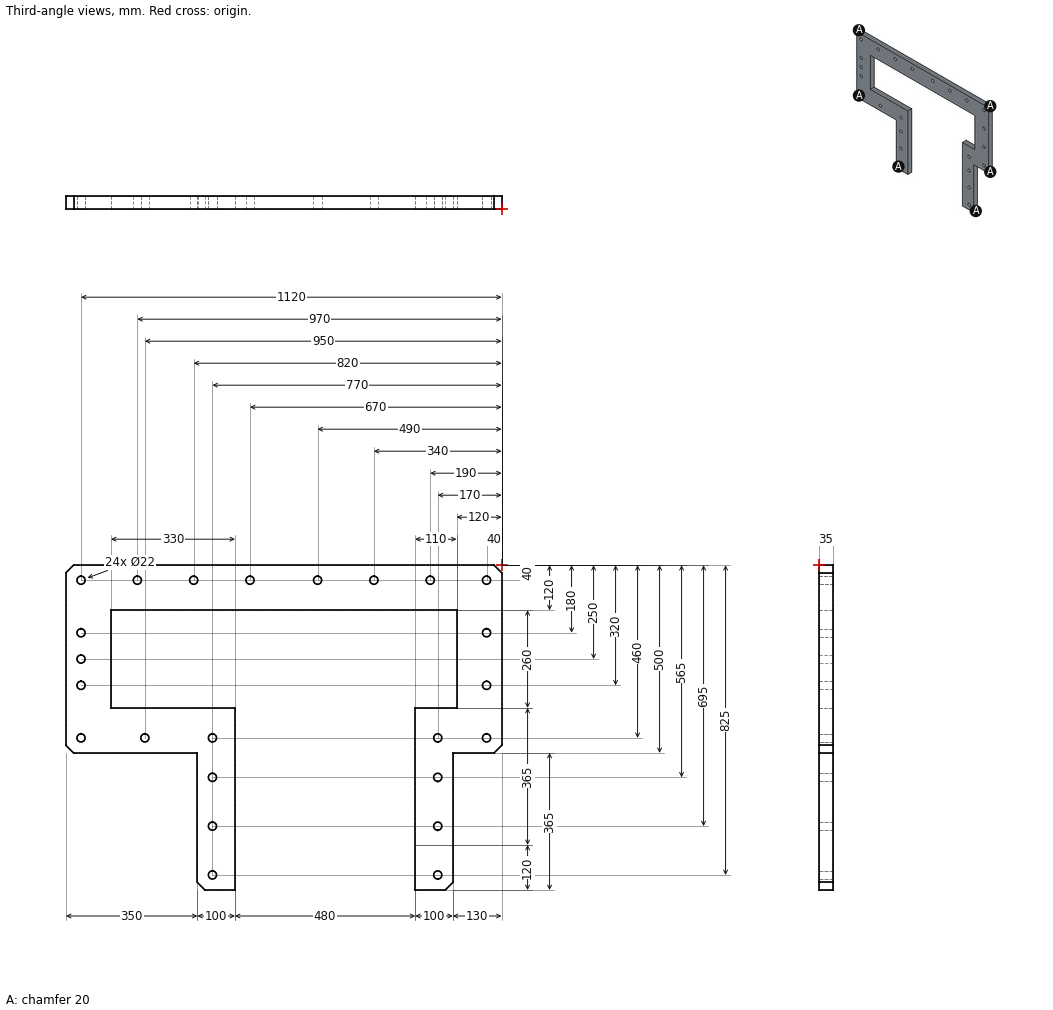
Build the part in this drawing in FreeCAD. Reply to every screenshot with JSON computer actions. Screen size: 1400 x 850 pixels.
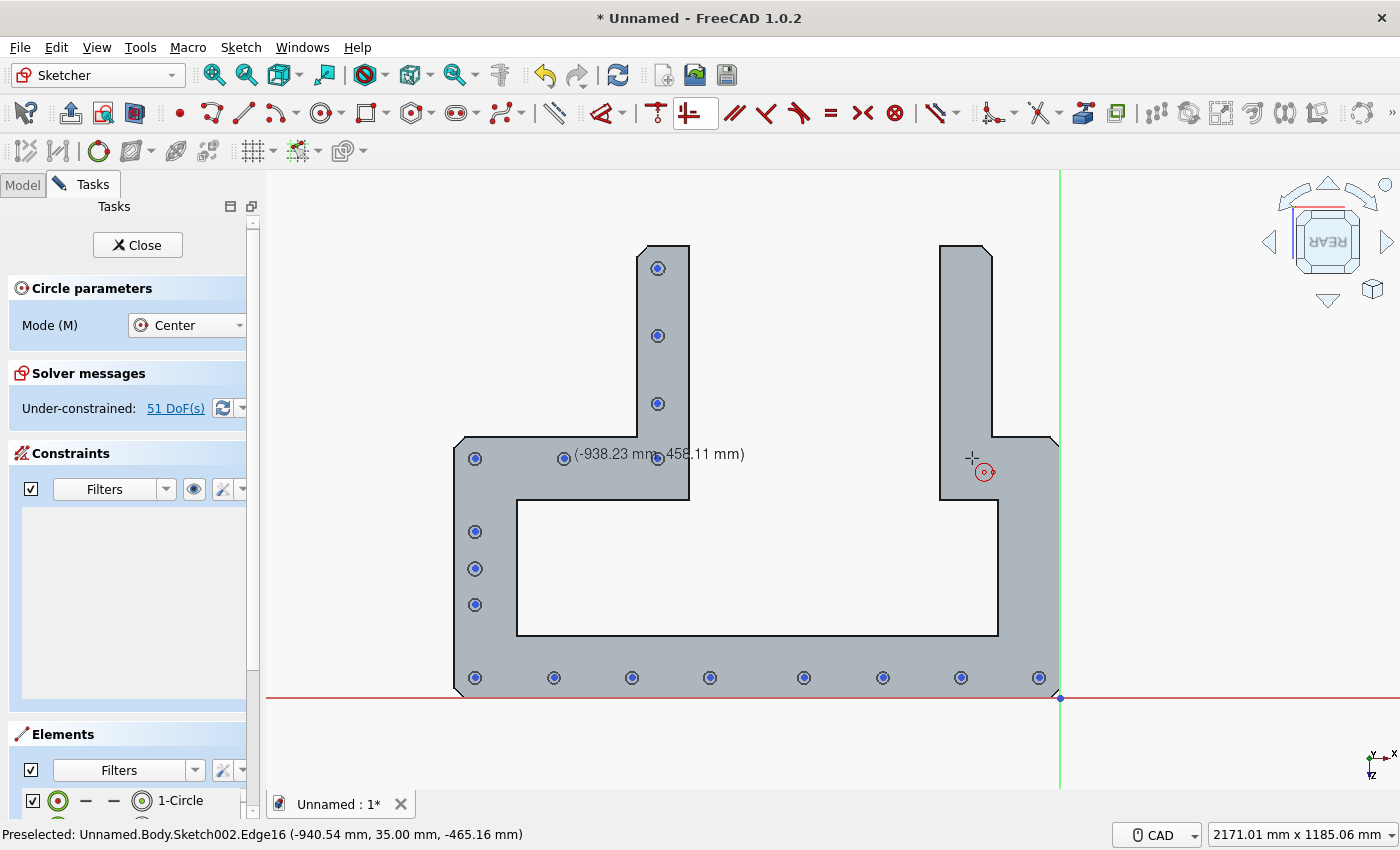
{"action": "left_click", "coordinate": [972, 458]}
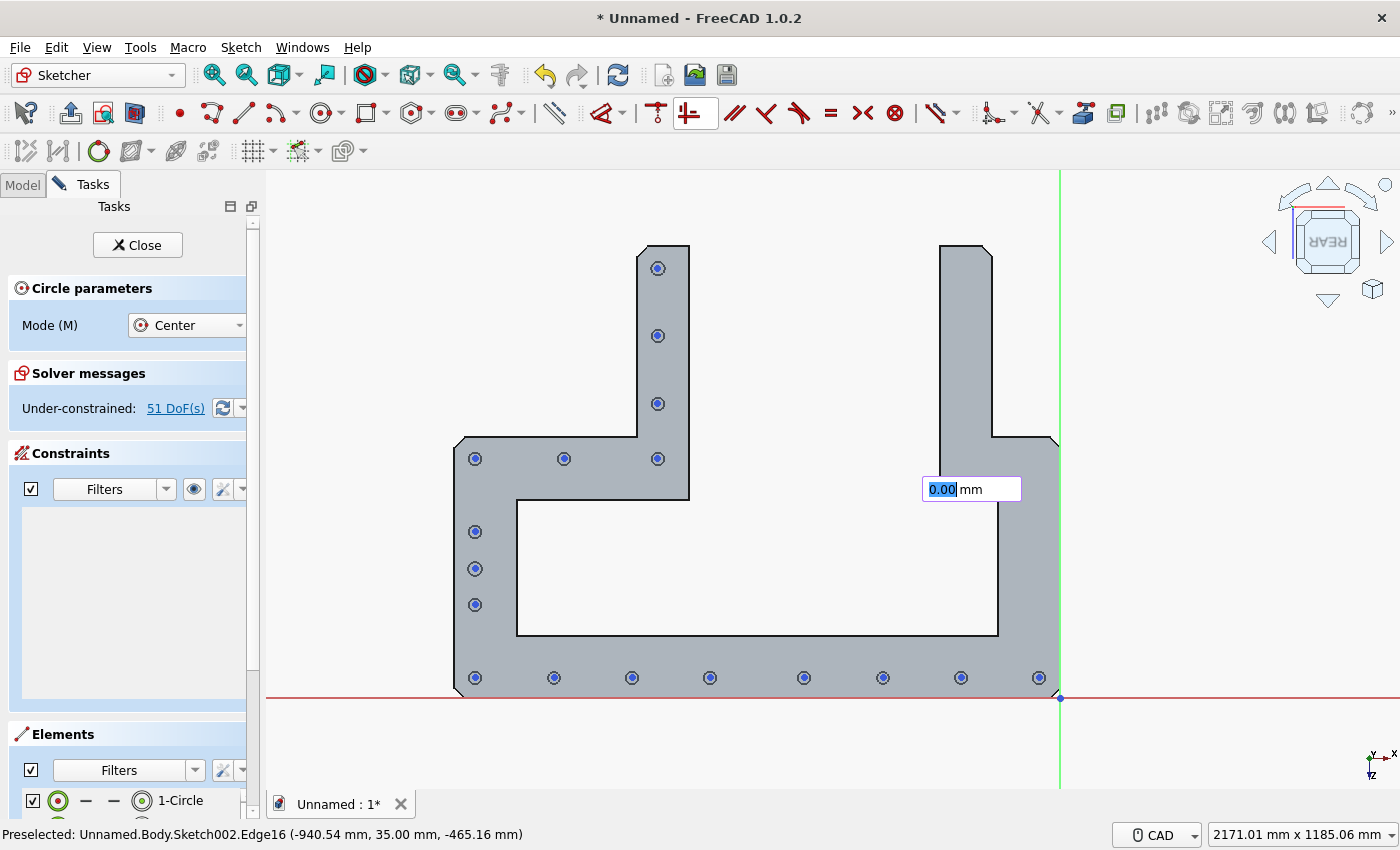
{"action": "scroll", "coordinate": [976, 454], "scroll_direction": "up", "scroll_amount": 6}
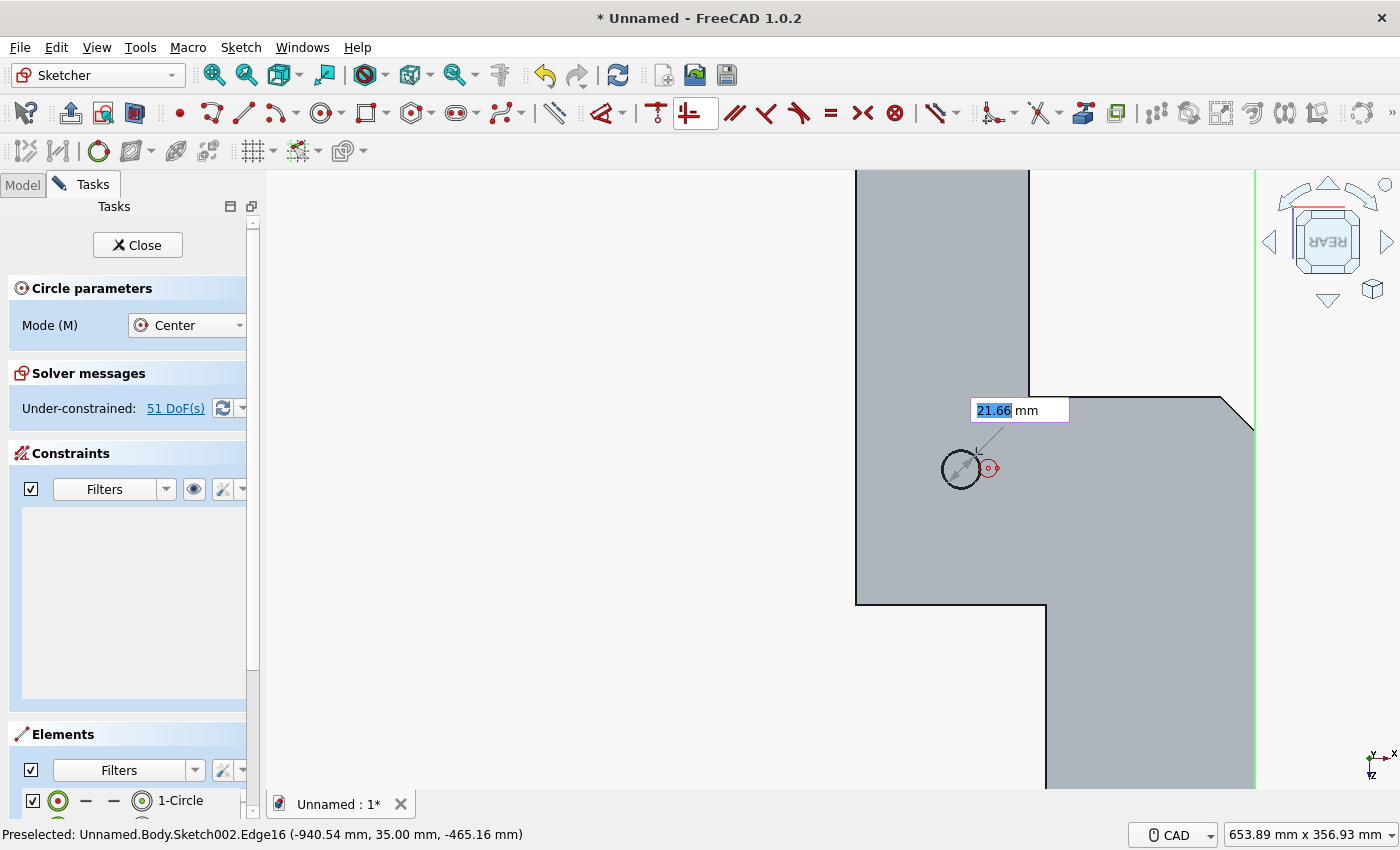
{"action": "left_click", "coordinate": [973, 453]}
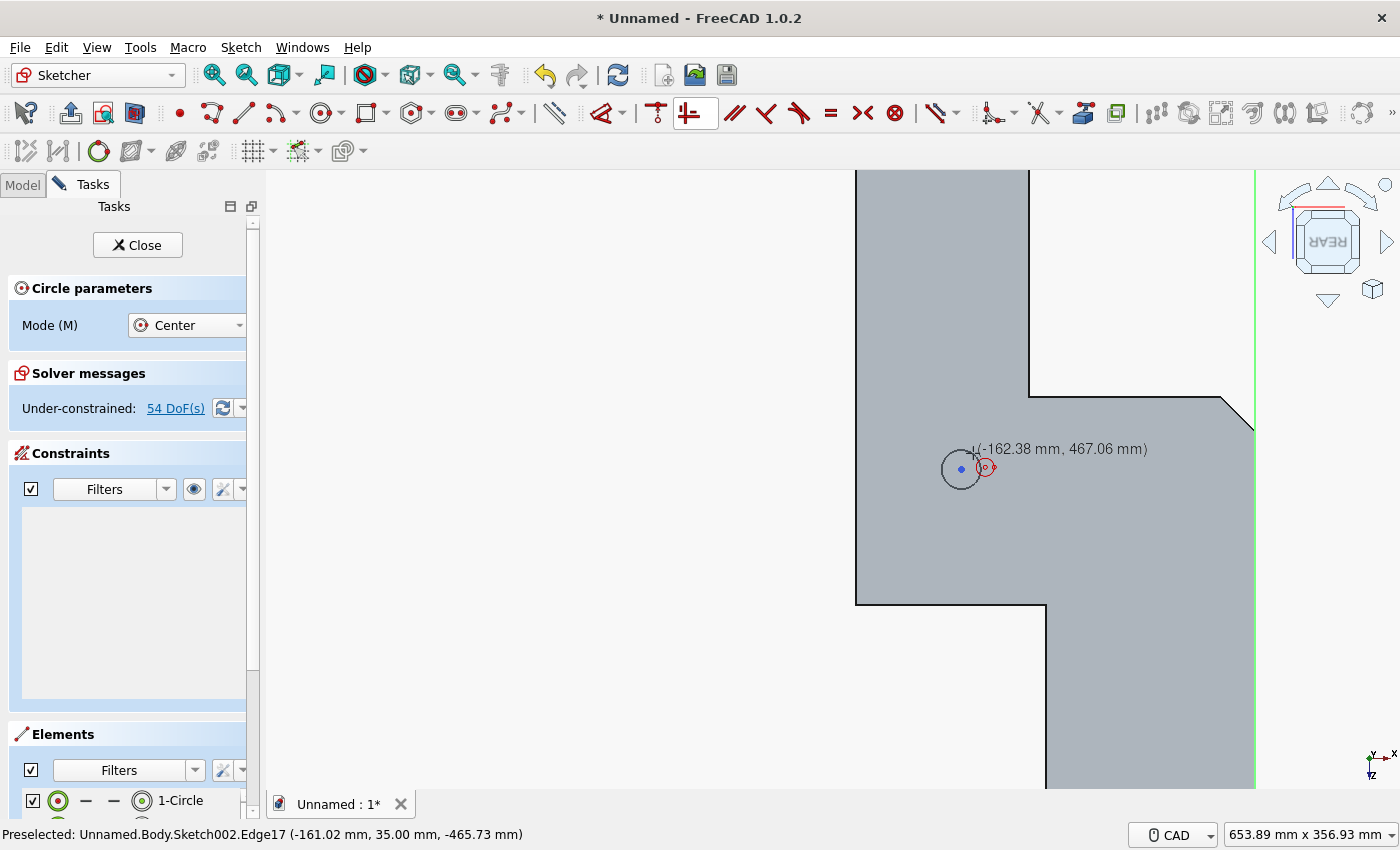
{"action": "scroll", "coordinate": [976, 454], "scroll_direction": "down", "scroll_amount": 6}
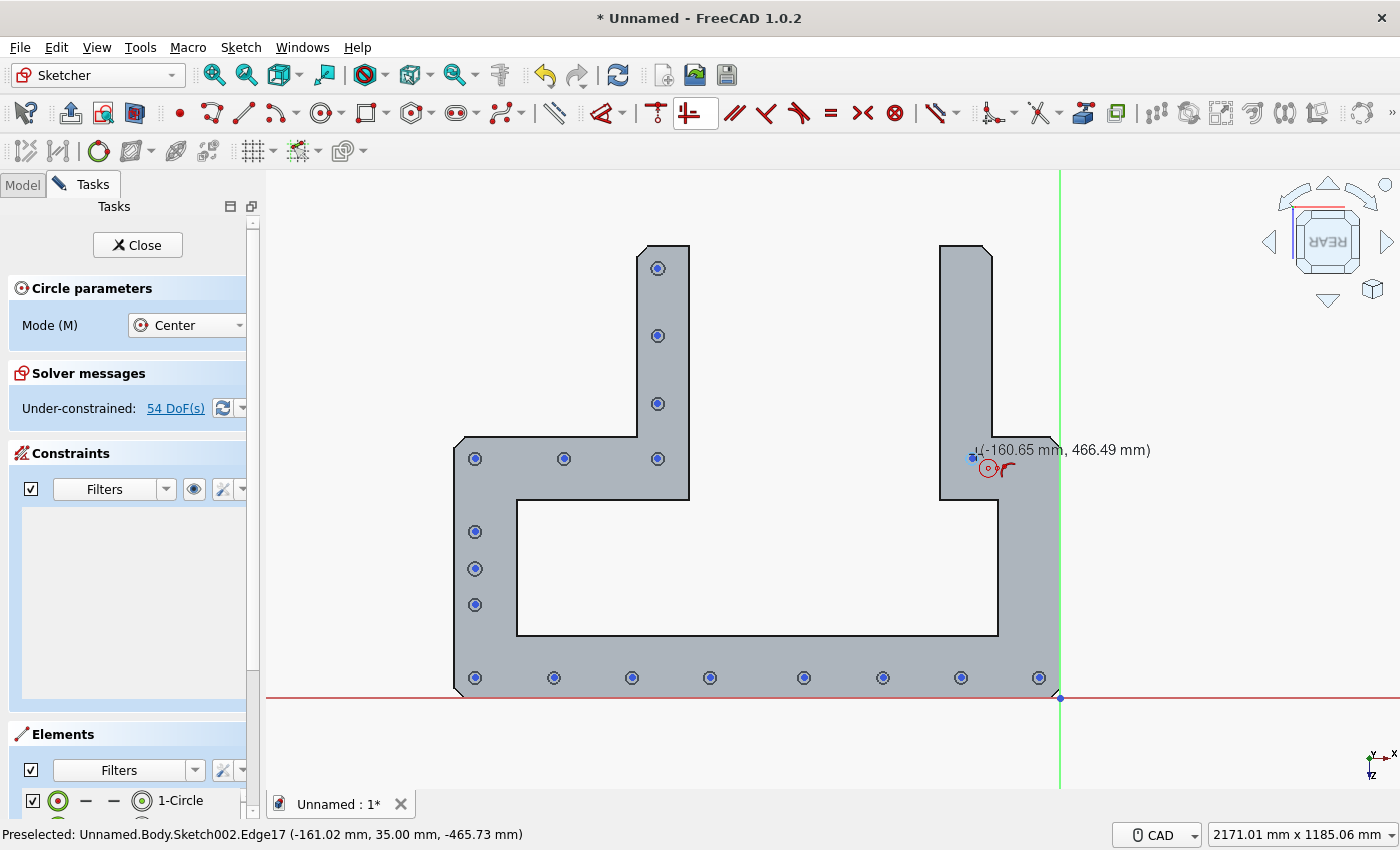
{"action": "left_click", "coordinate": [972, 403]}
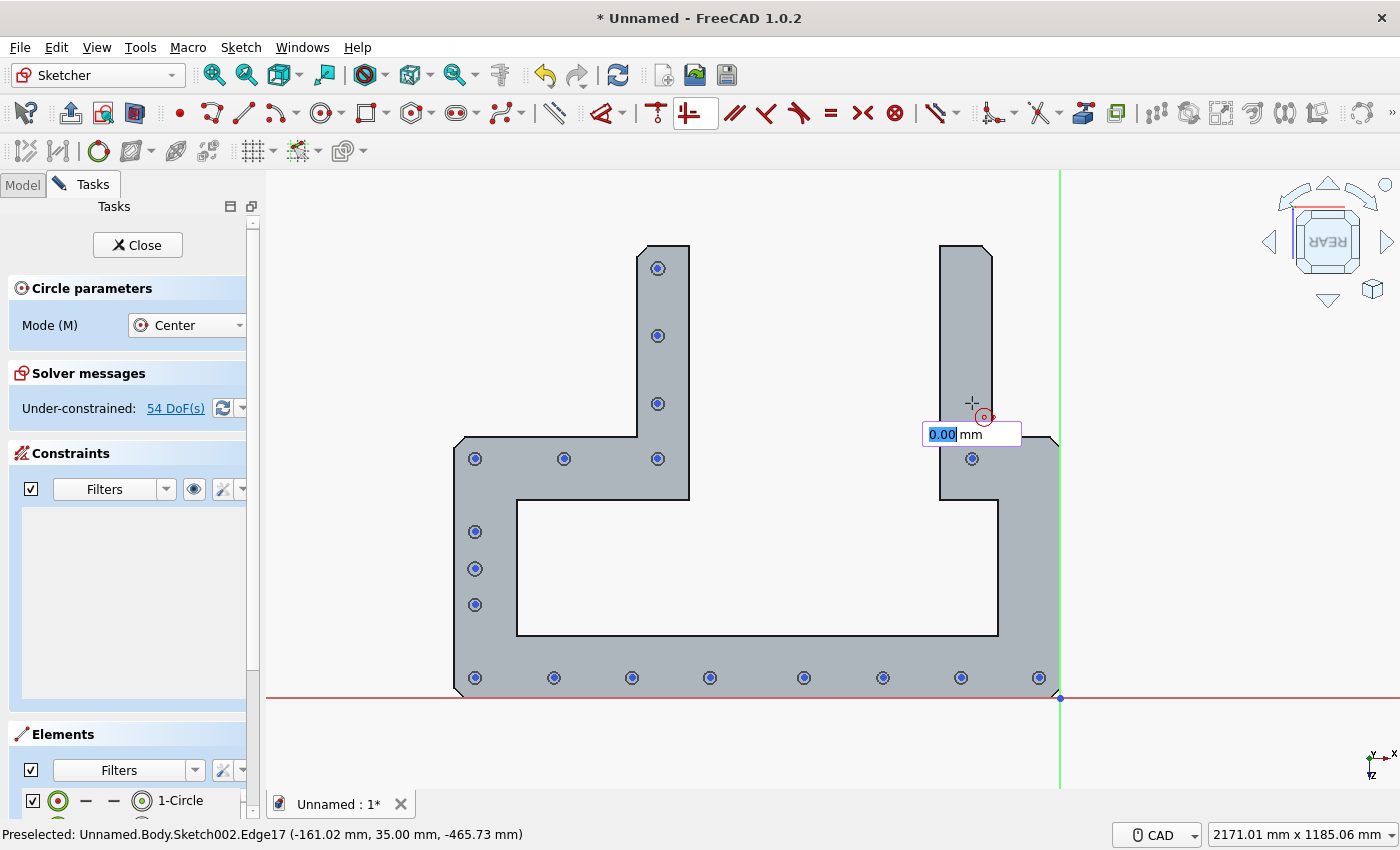
{"action": "scroll", "coordinate": [976, 399], "scroll_direction": "up", "scroll_amount": 6}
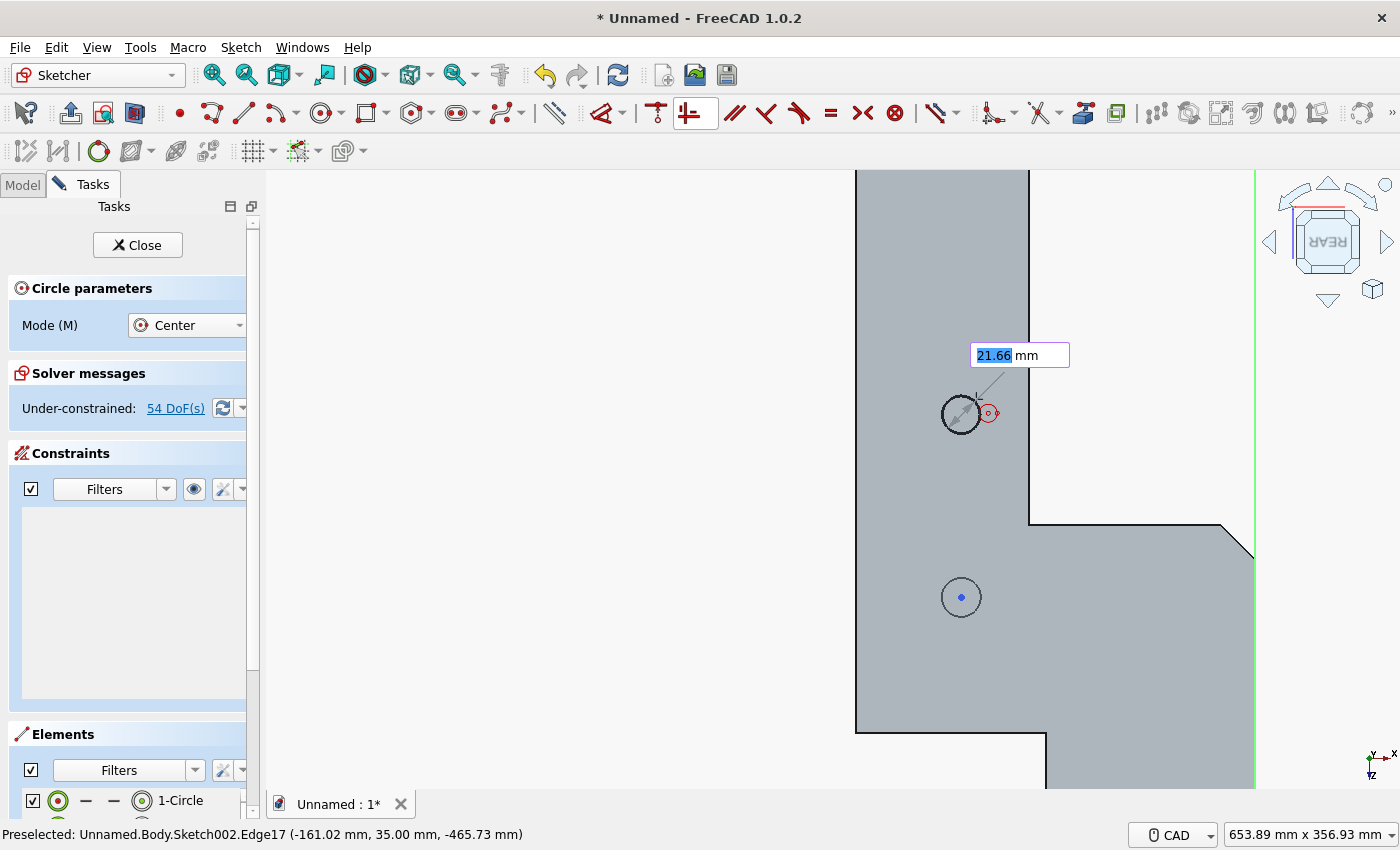
{"action": "left_click", "coordinate": [973, 398]}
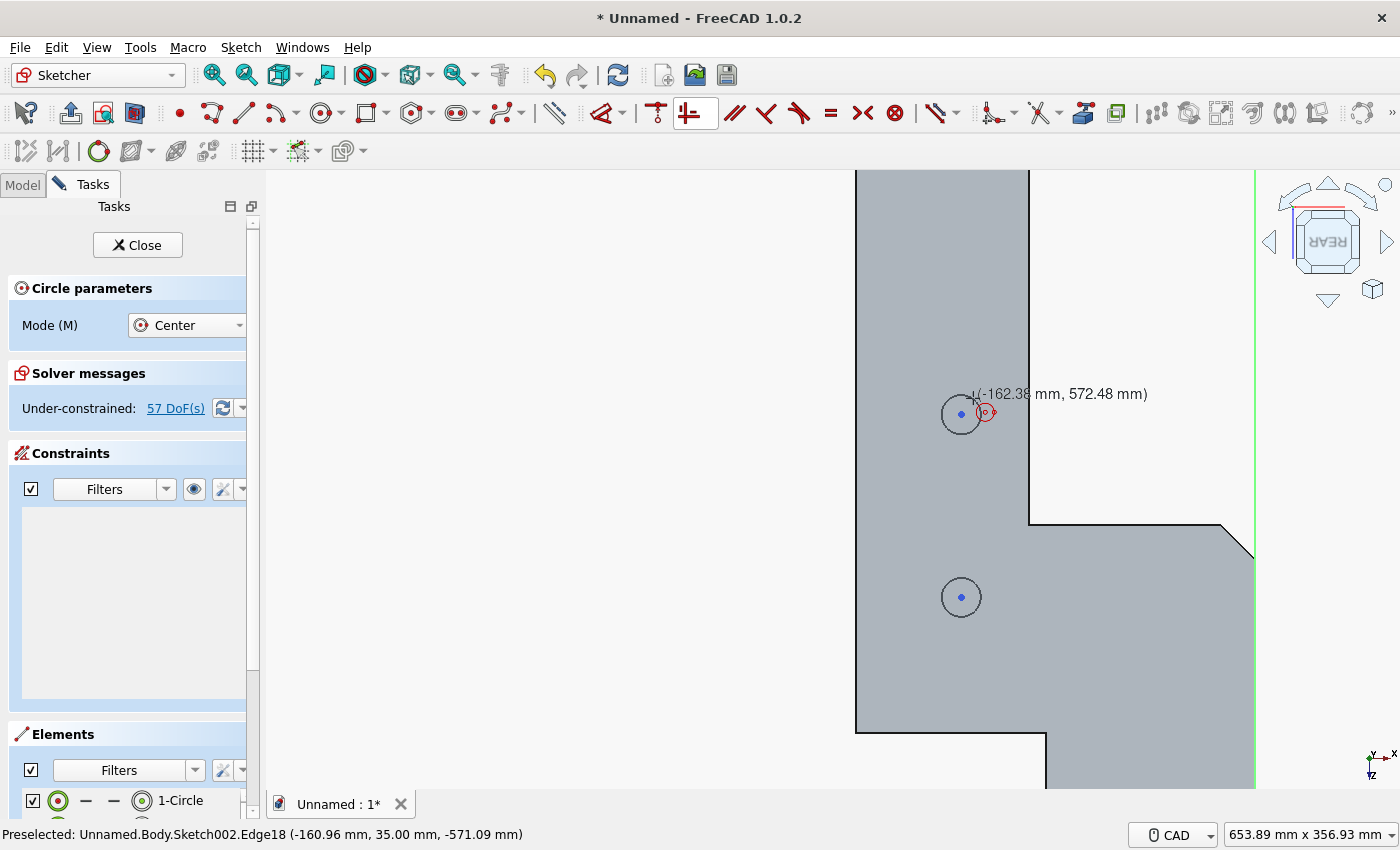
{"action": "scroll", "coordinate": [976, 399], "scroll_direction": "down", "scroll_amount": 6}